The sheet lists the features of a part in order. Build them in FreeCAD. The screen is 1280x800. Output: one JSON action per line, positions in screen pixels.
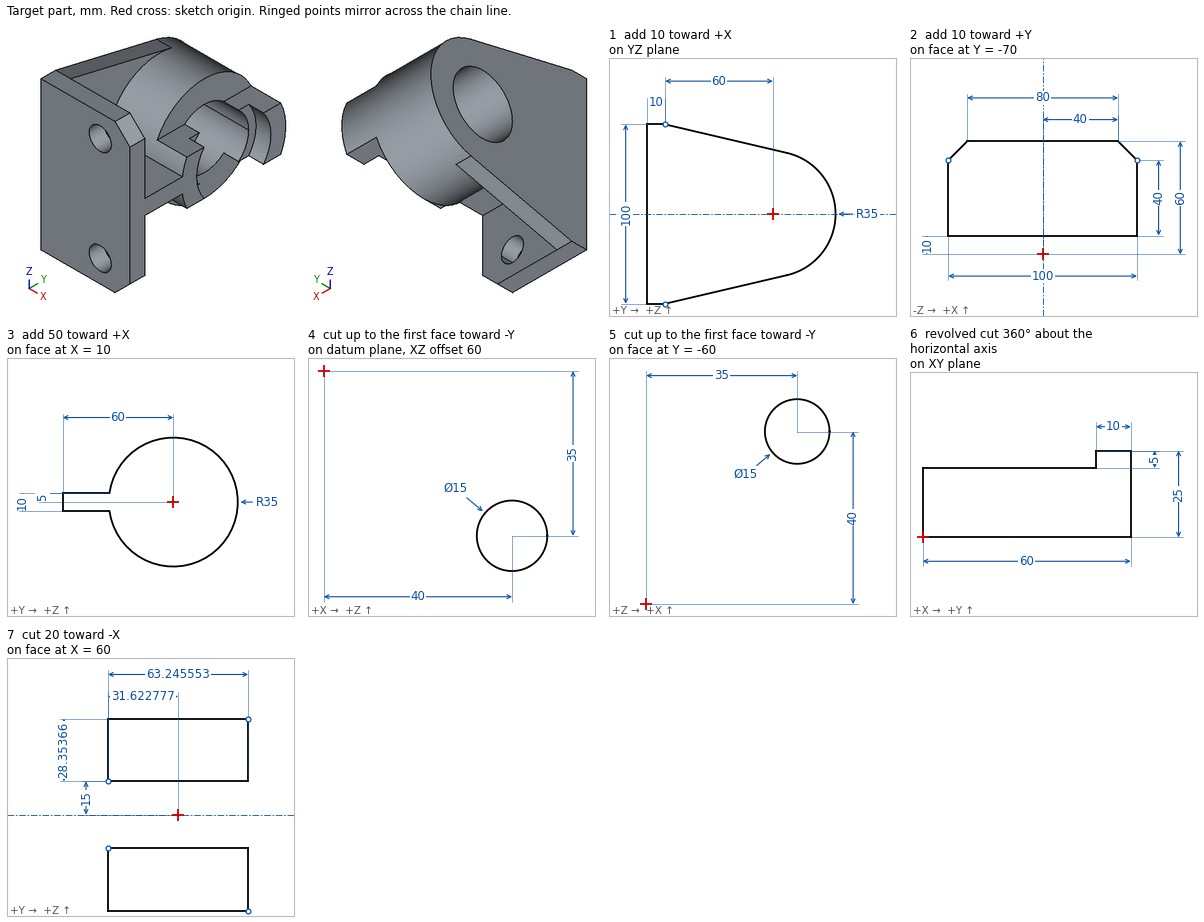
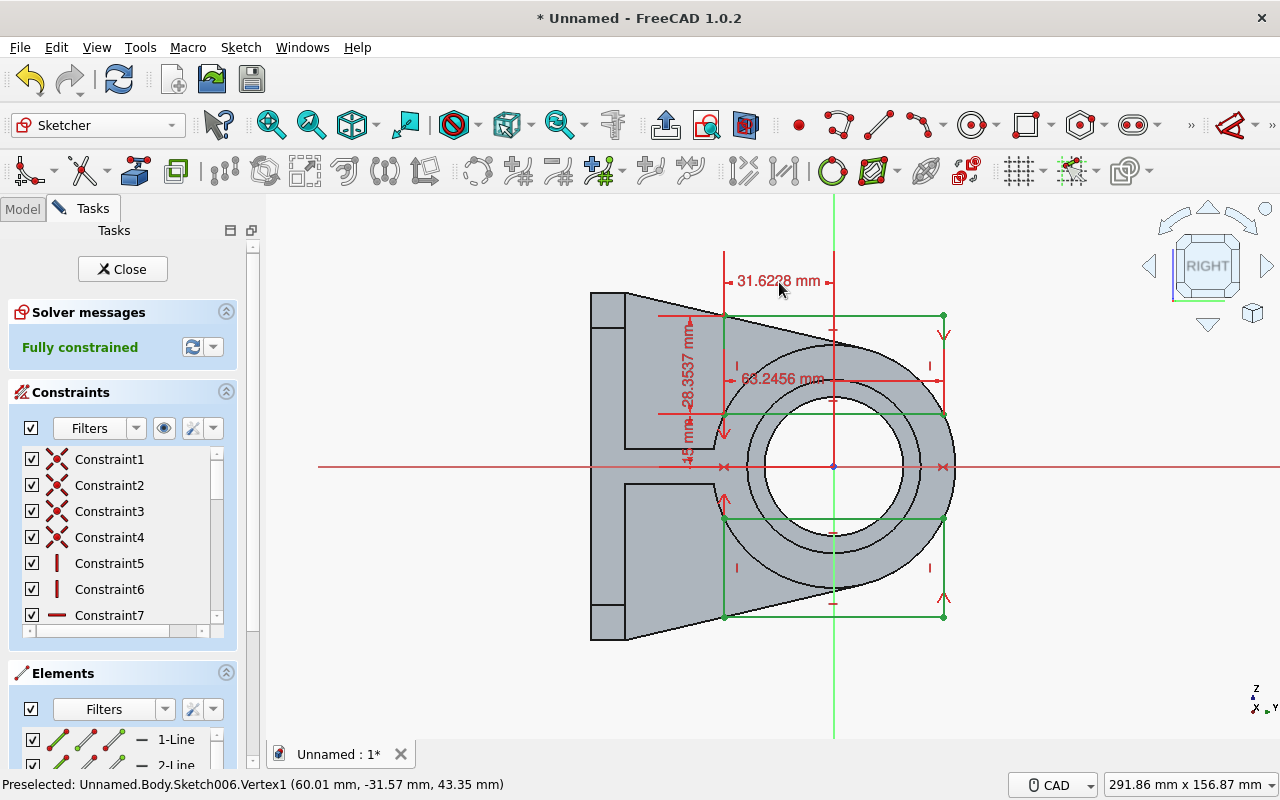
{"action": "left_click", "coordinate": [123, 269]}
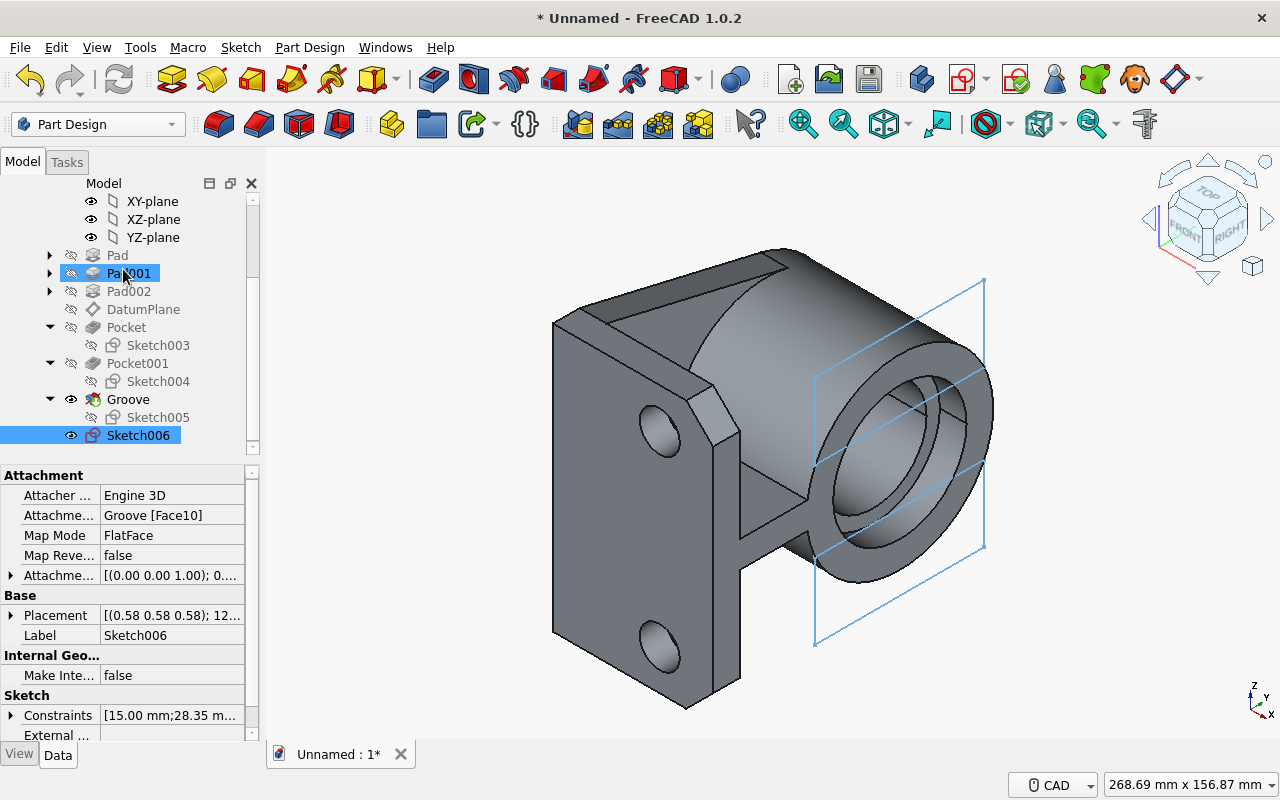
{"action": "left_click", "coordinate": [434, 80]}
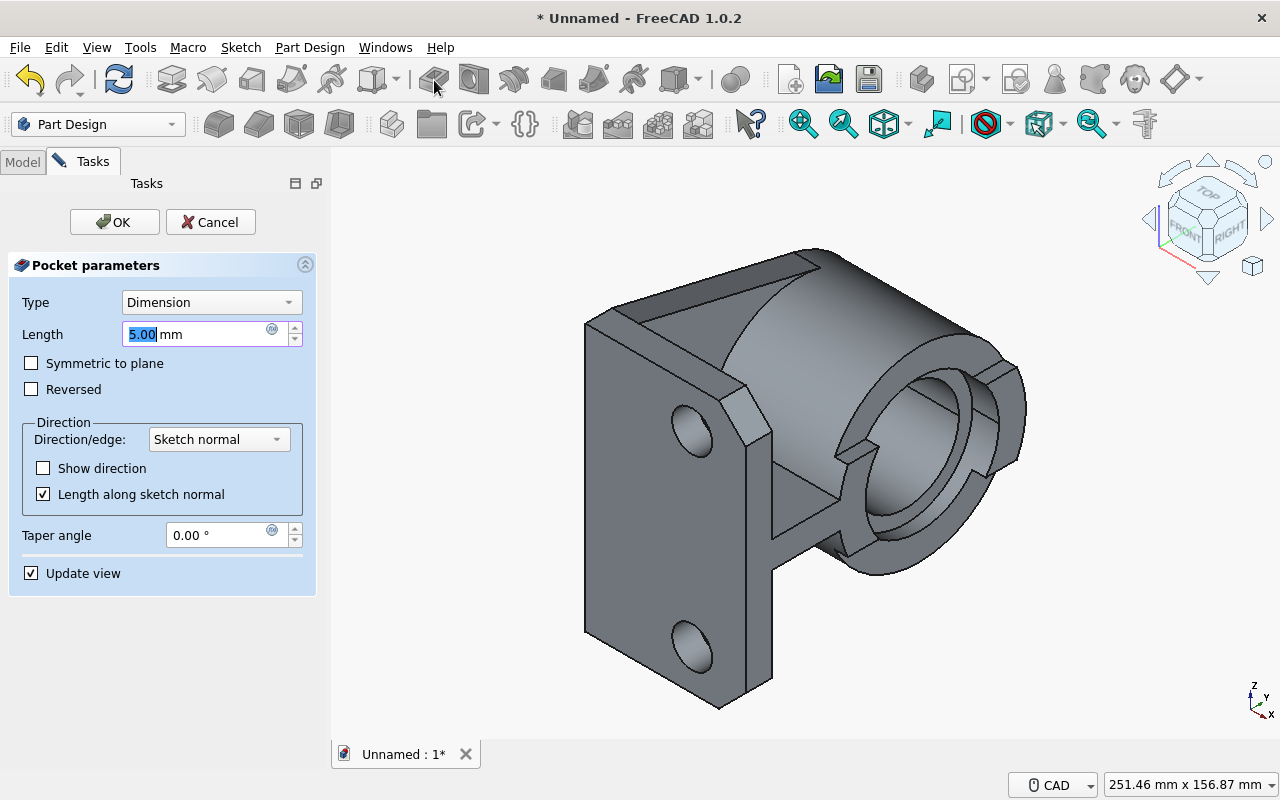
{"action": "type", "text": "20"}
{"action": "key", "text": "Tab"}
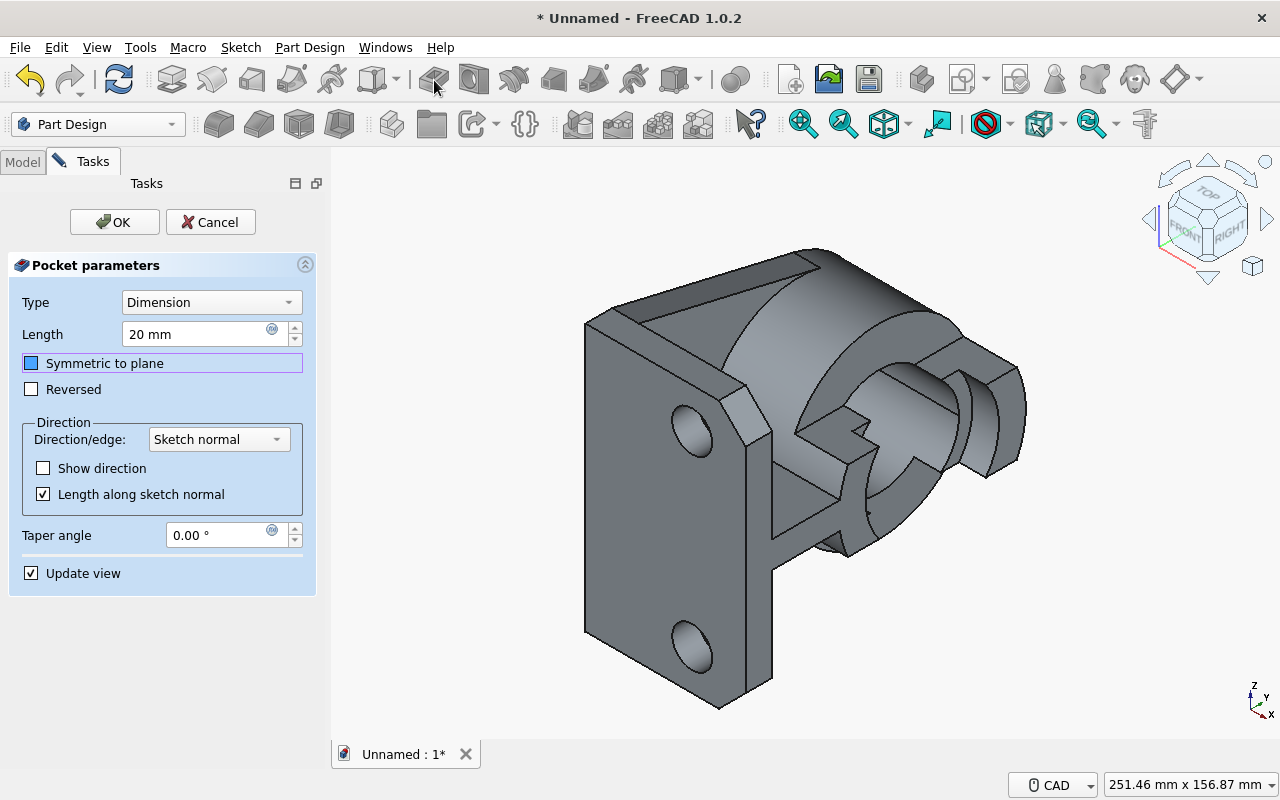
{"action": "left_click", "coordinate": [115, 222]}